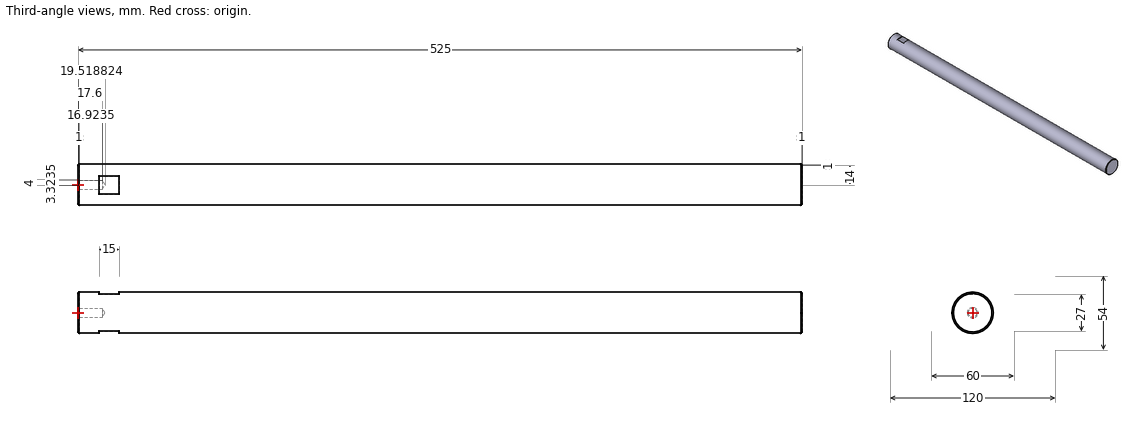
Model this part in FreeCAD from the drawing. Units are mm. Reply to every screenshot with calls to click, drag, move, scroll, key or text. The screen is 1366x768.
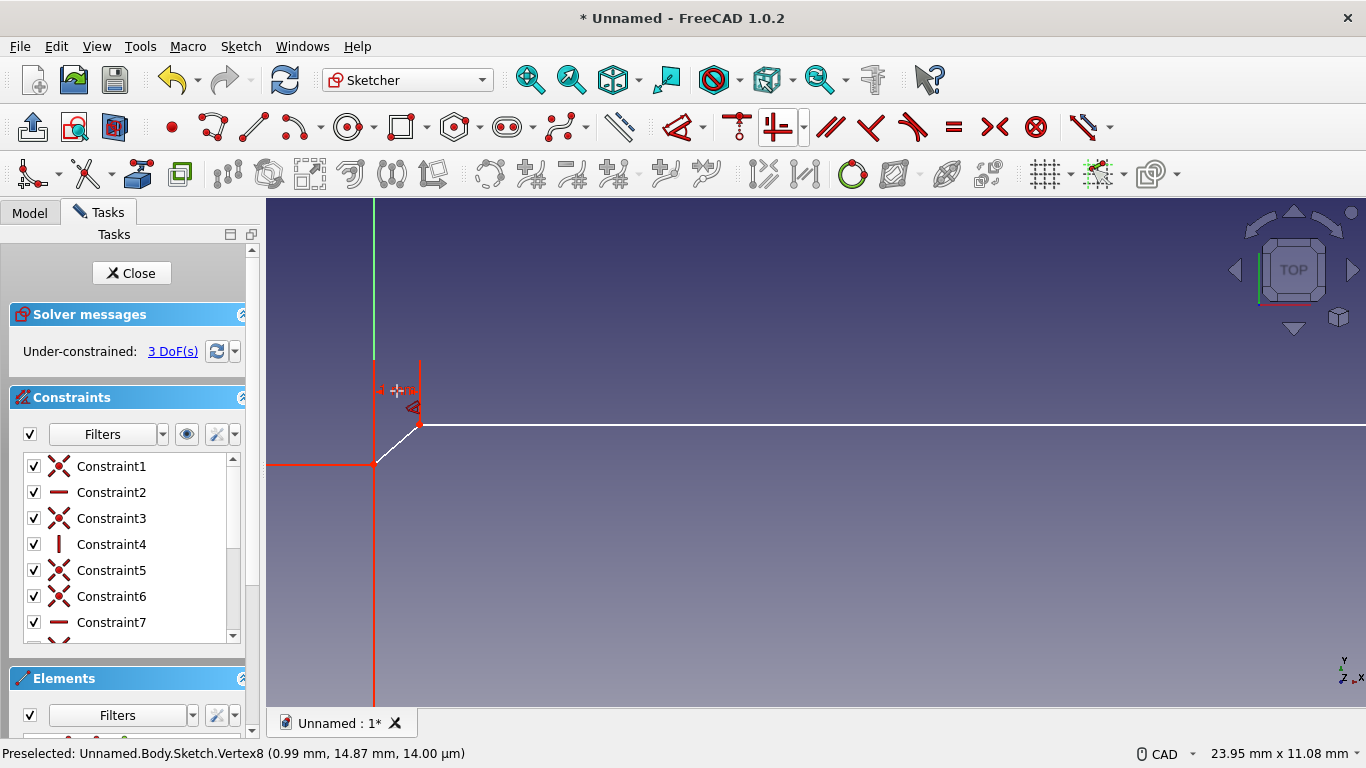
scroll(344, 442, down, 17)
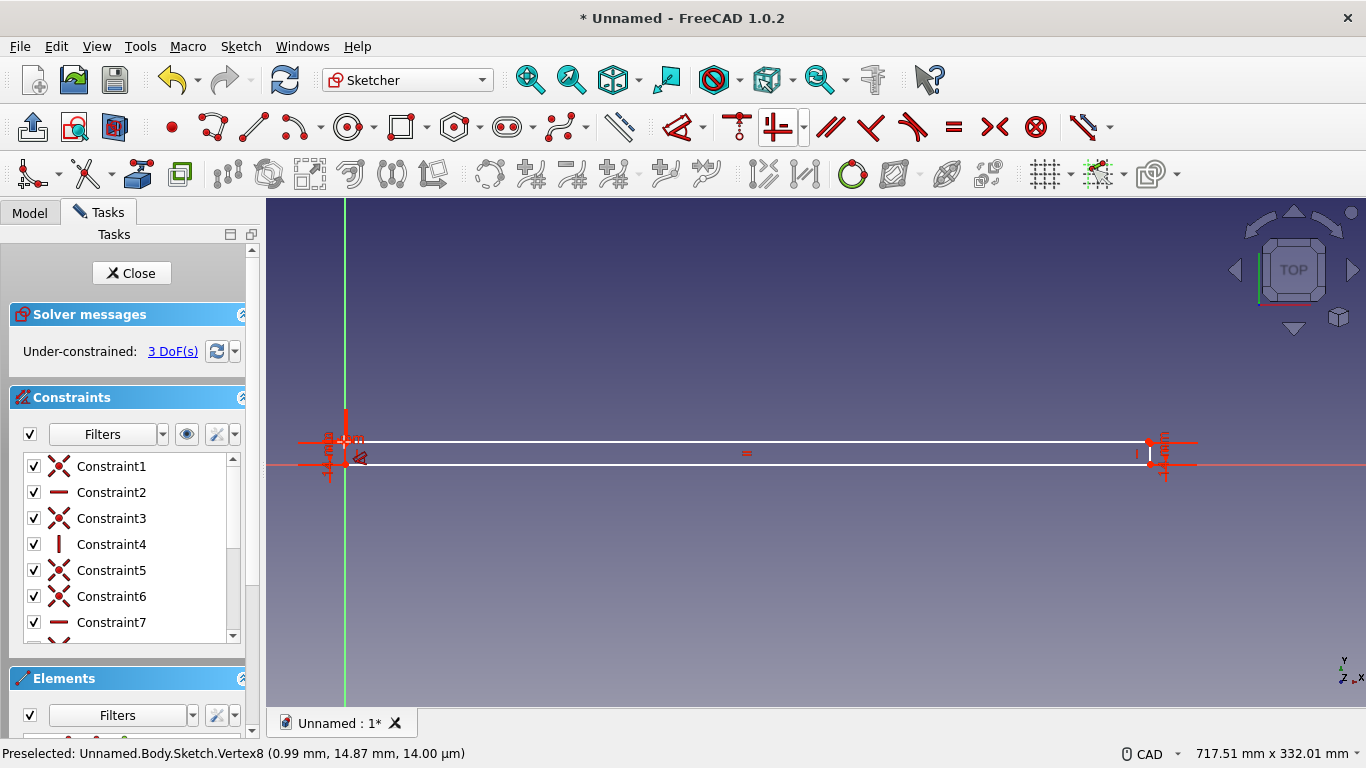
scroll(1150, 443, up, 17)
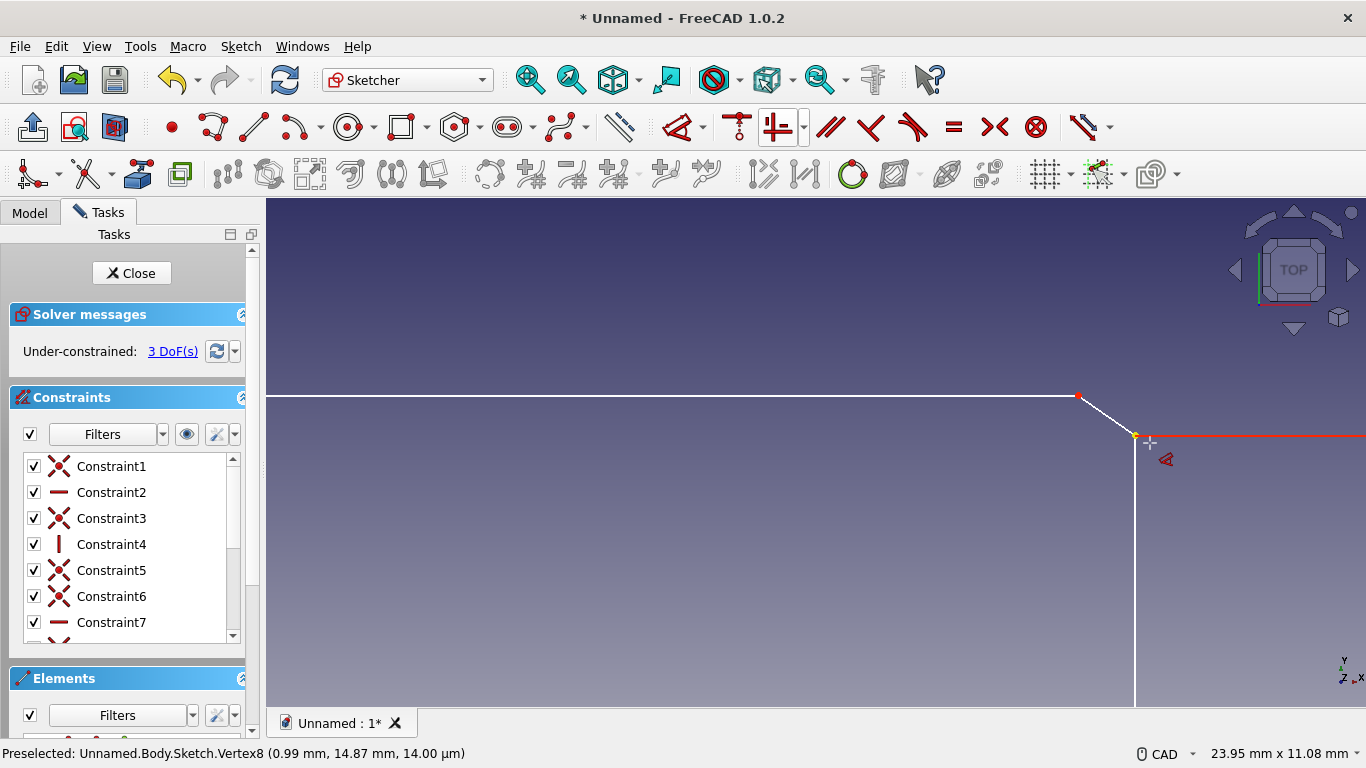
click(1118, 424)
click(1107, 362)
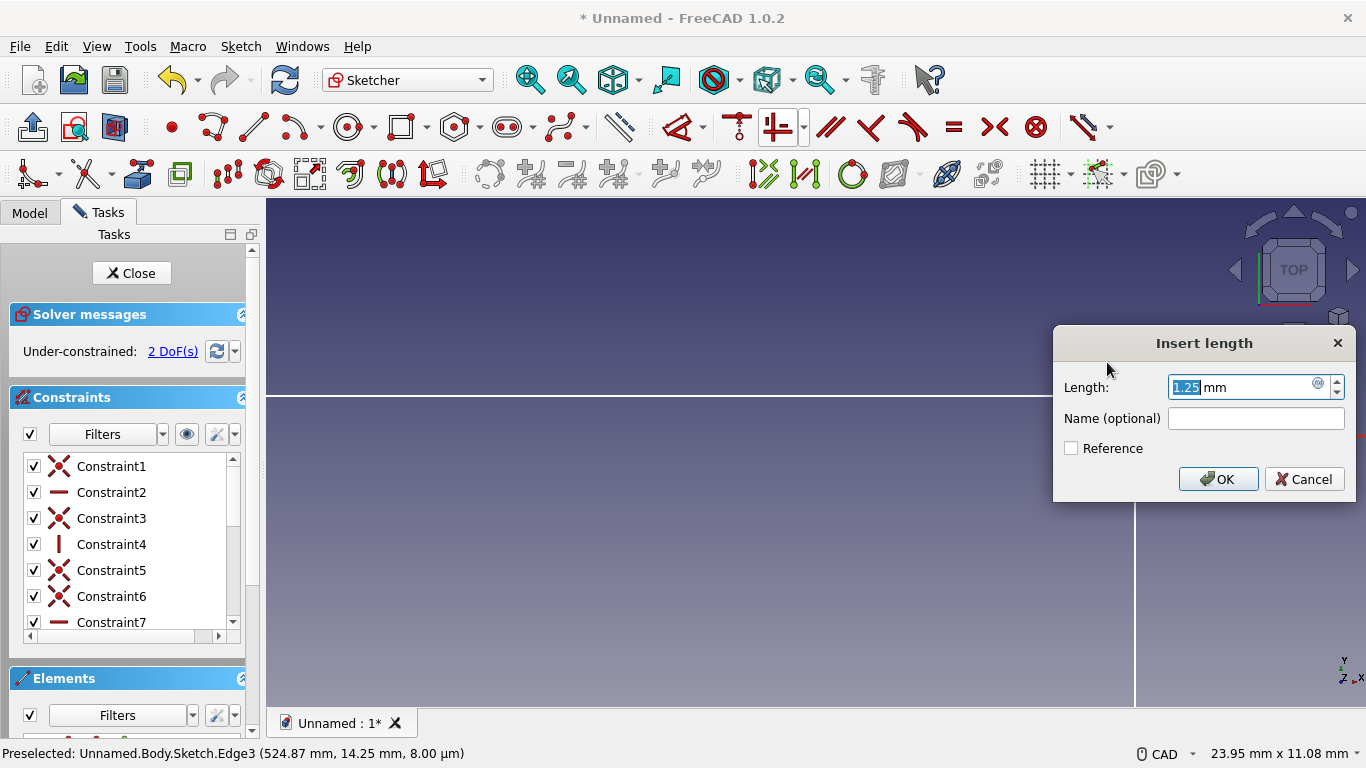
text(1)
key(Return)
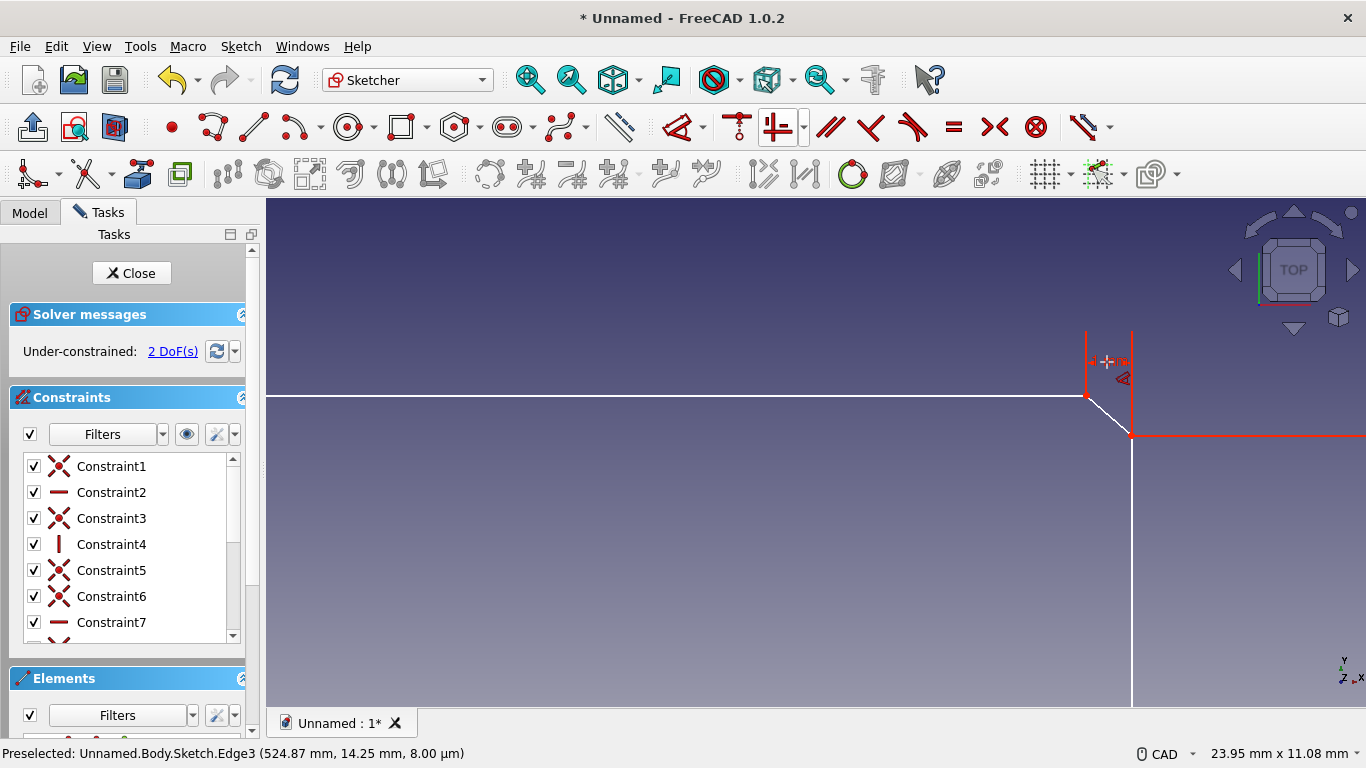
click(1118, 424)
click(1166, 416)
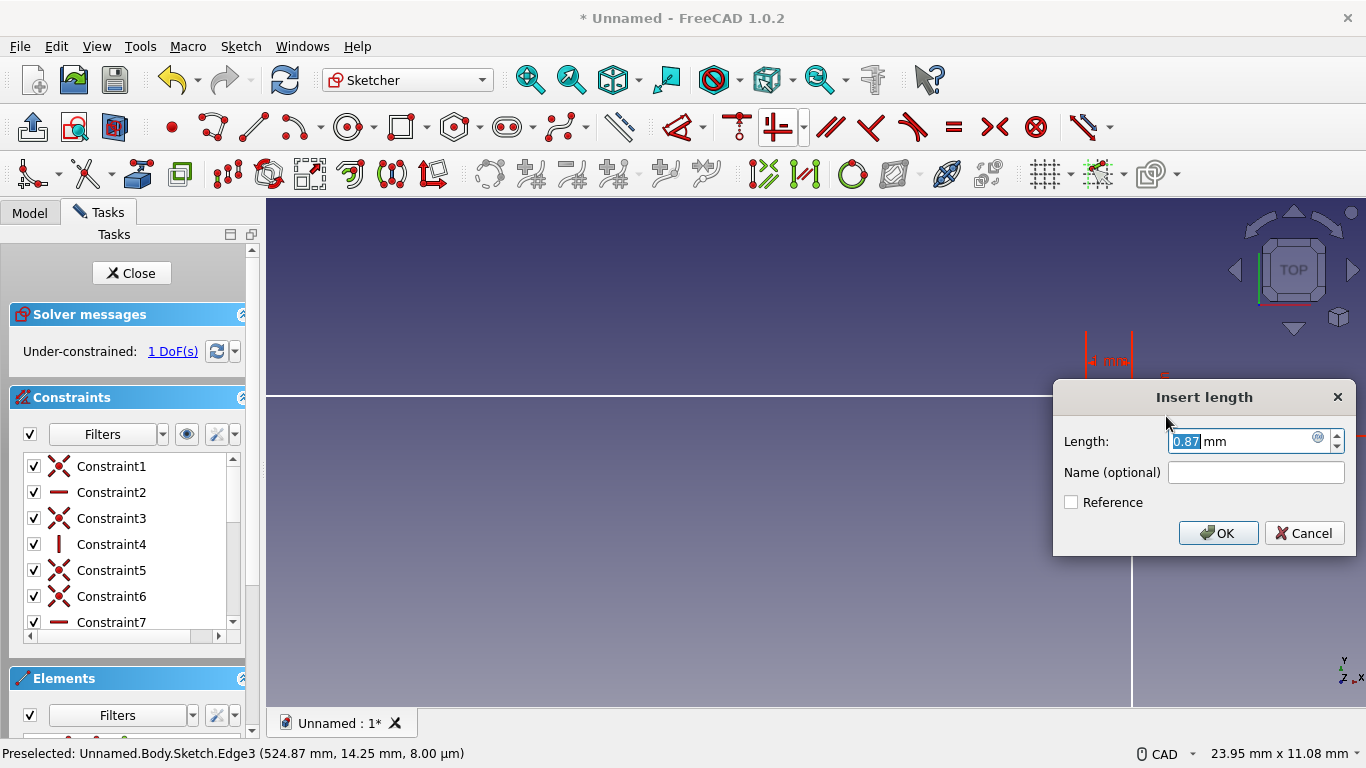
text(1)
key(Return)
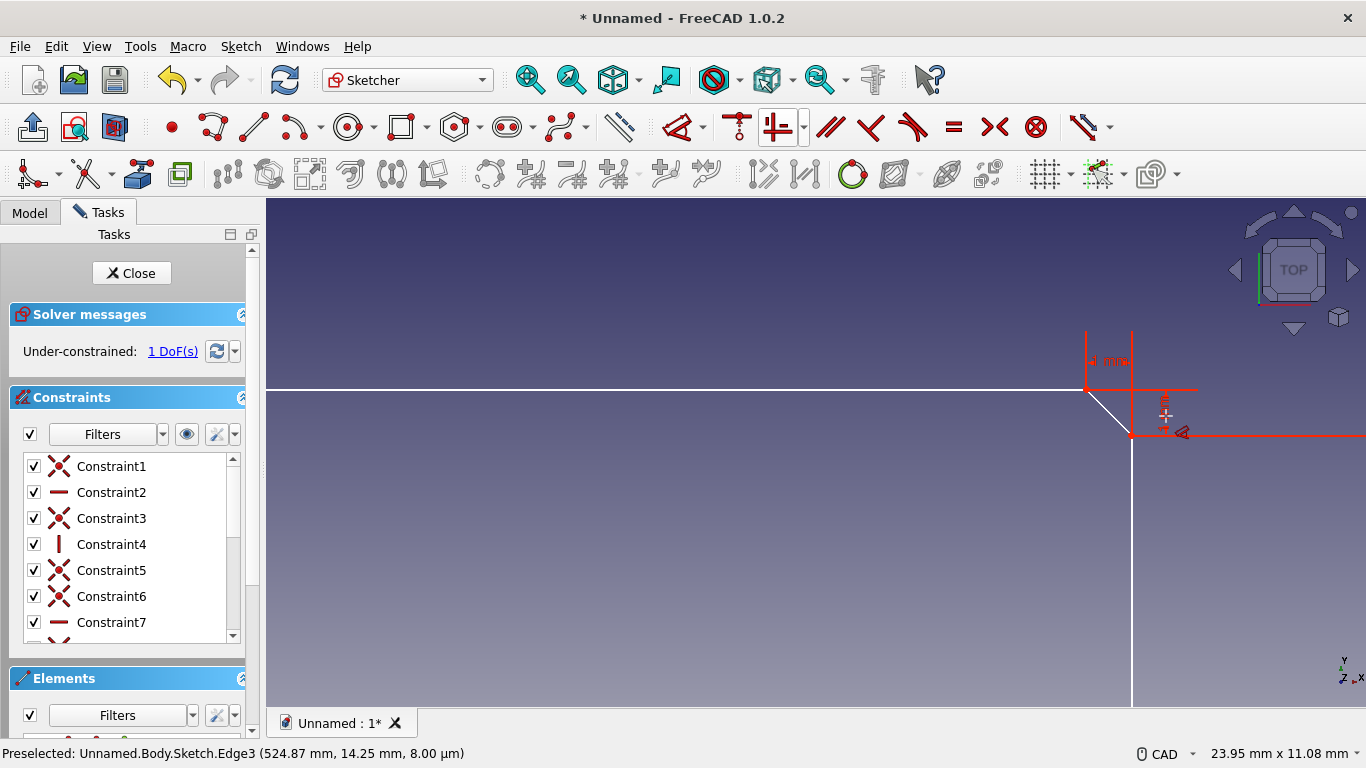
scroll(1151, 443, down, 17)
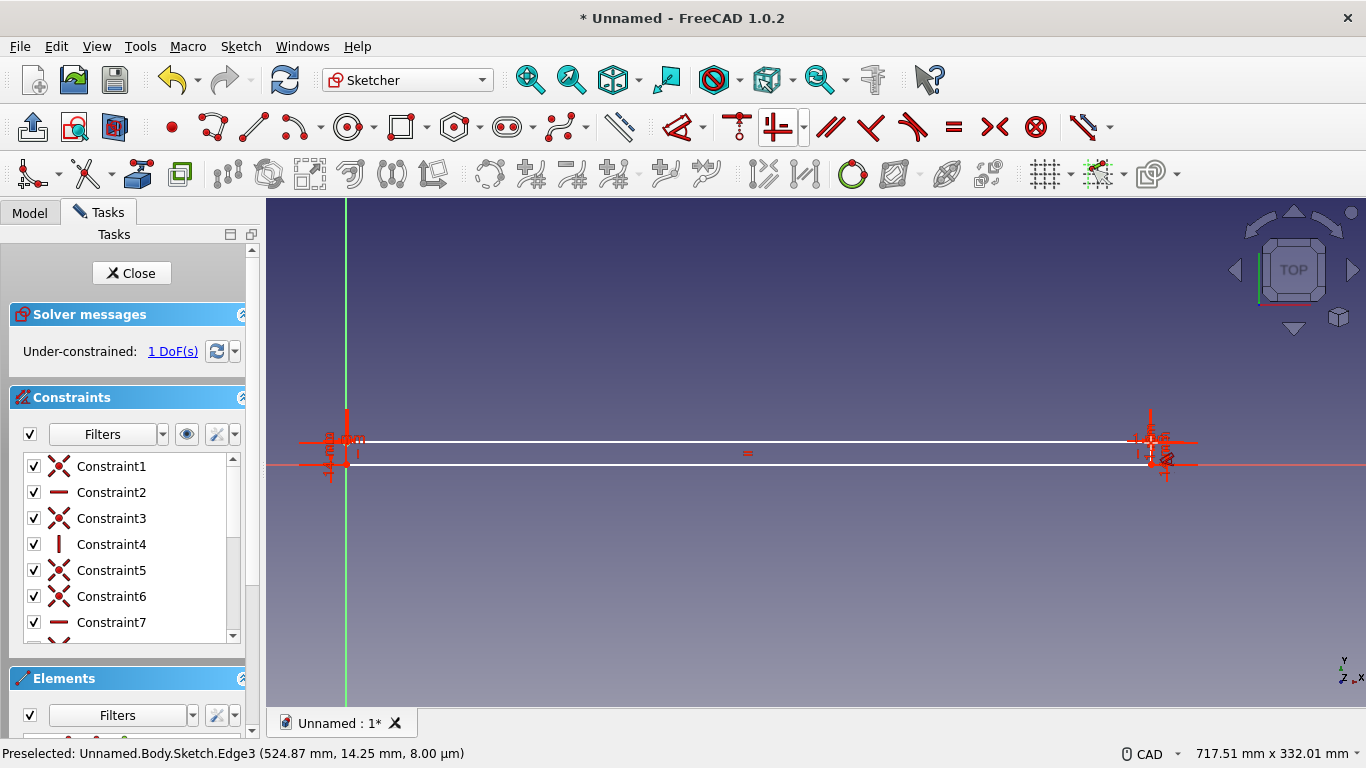
click(588, 465)
click(749, 499)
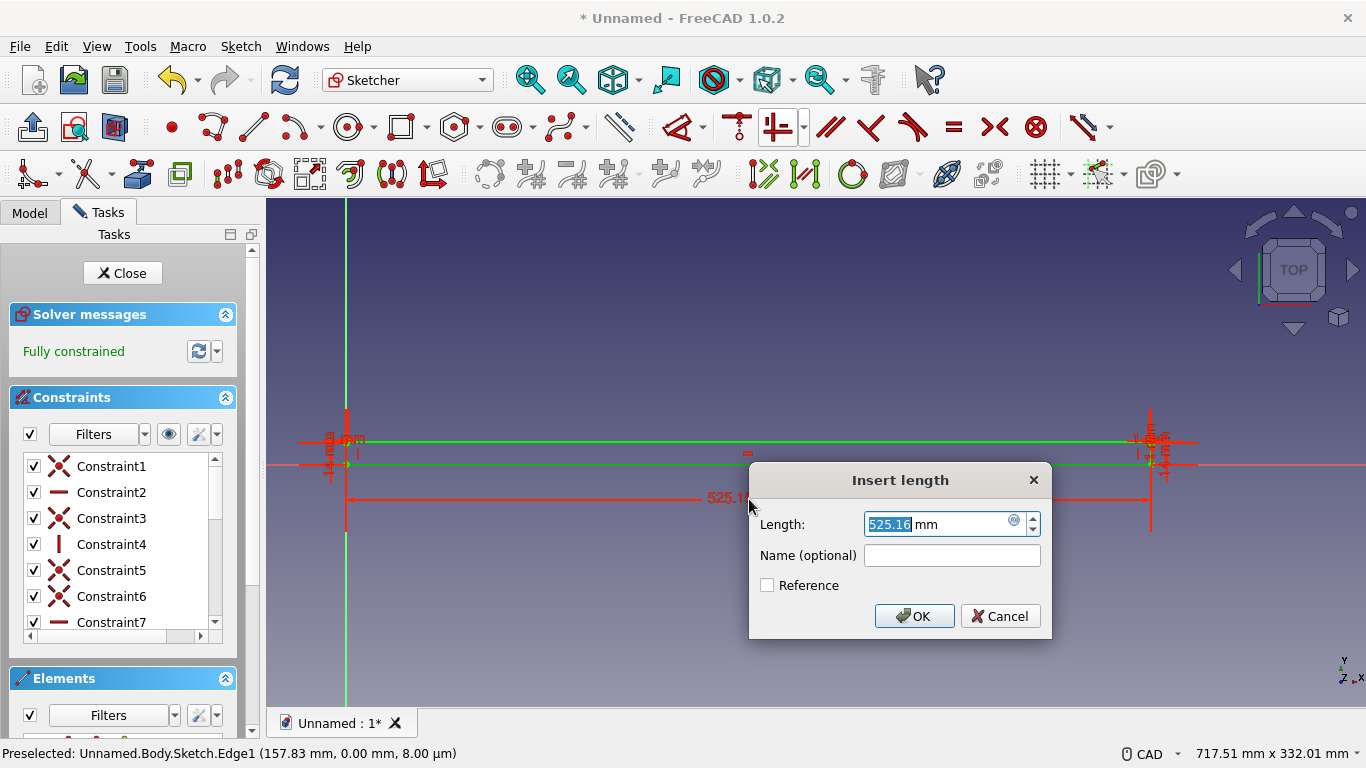
text(525)
key(Return)
key(Escape)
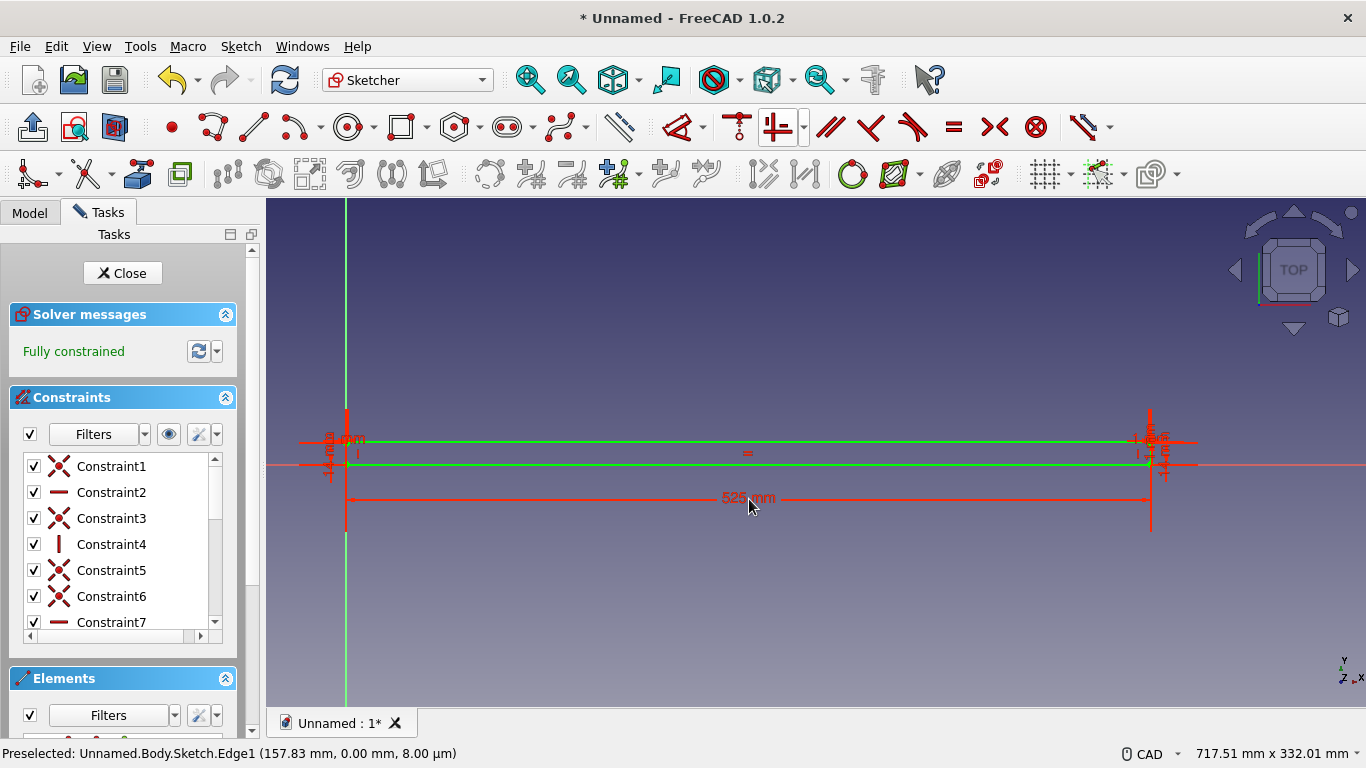
click(123, 273)